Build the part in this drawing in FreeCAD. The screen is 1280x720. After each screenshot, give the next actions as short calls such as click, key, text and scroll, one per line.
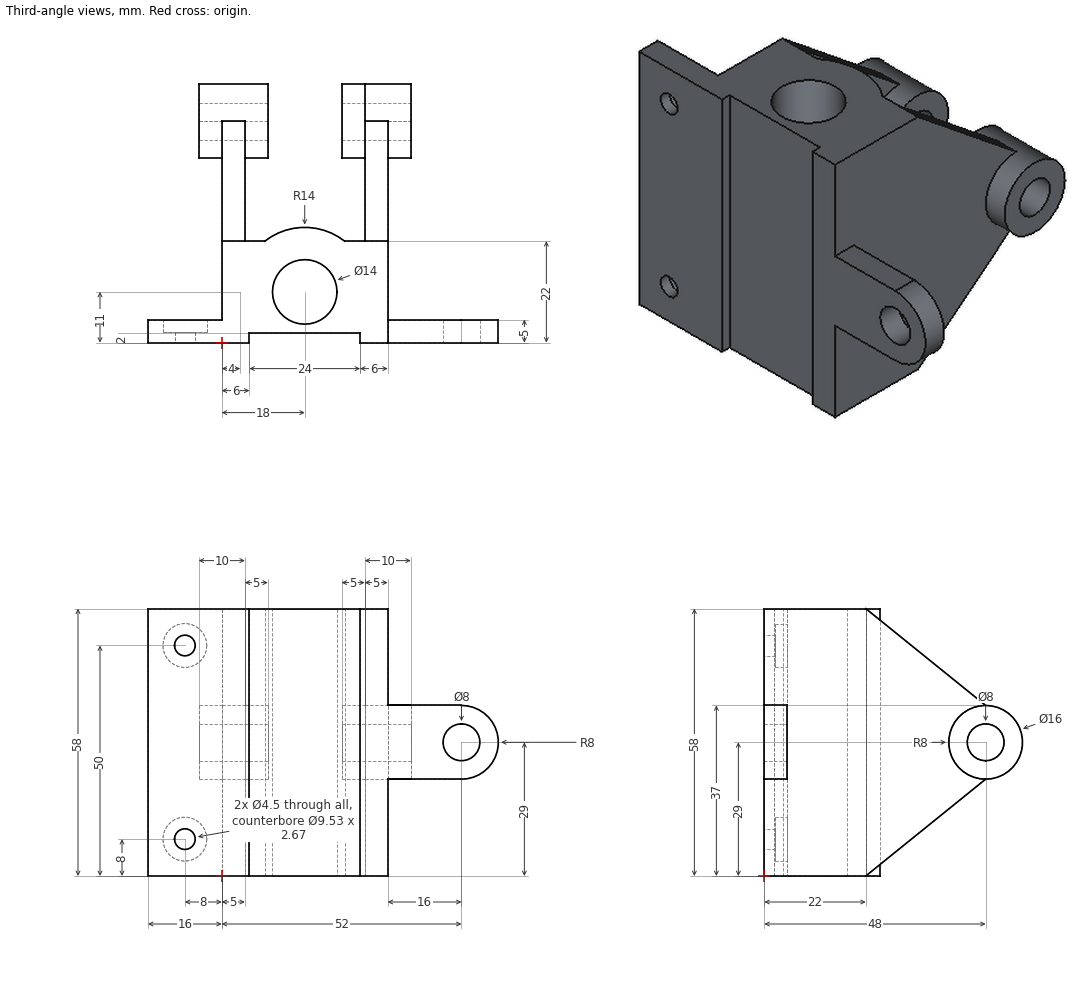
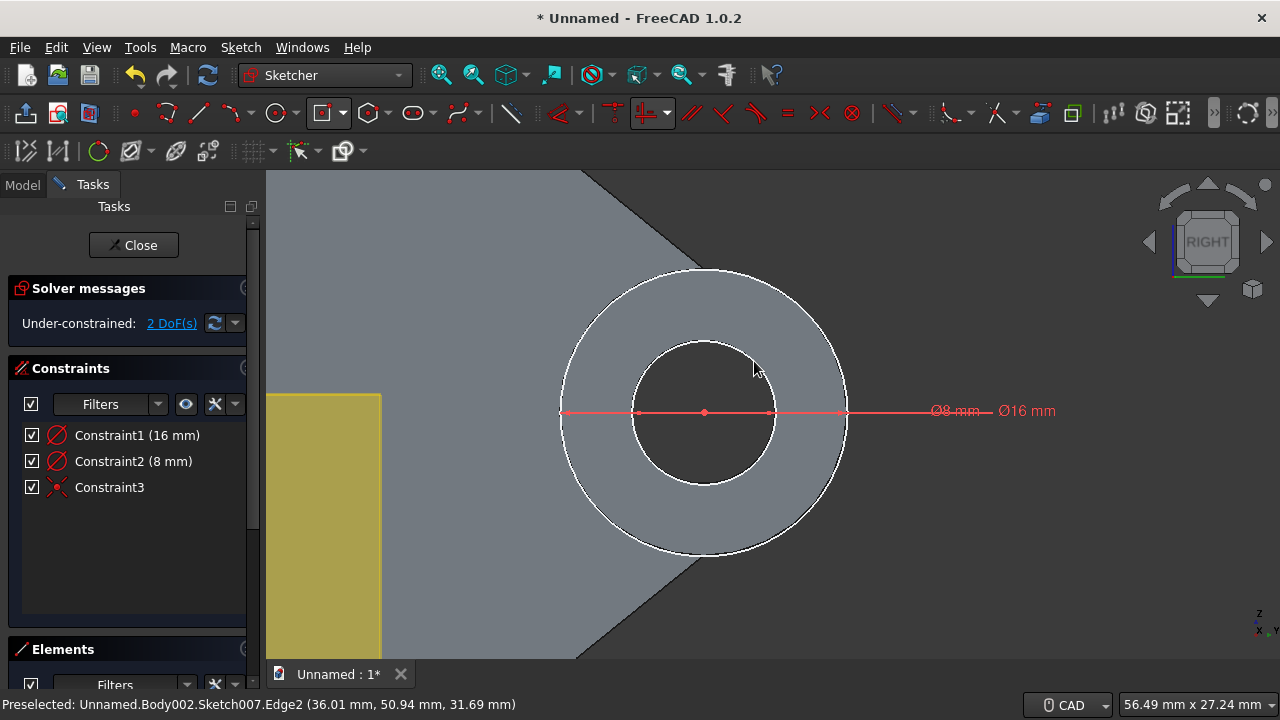
key(d)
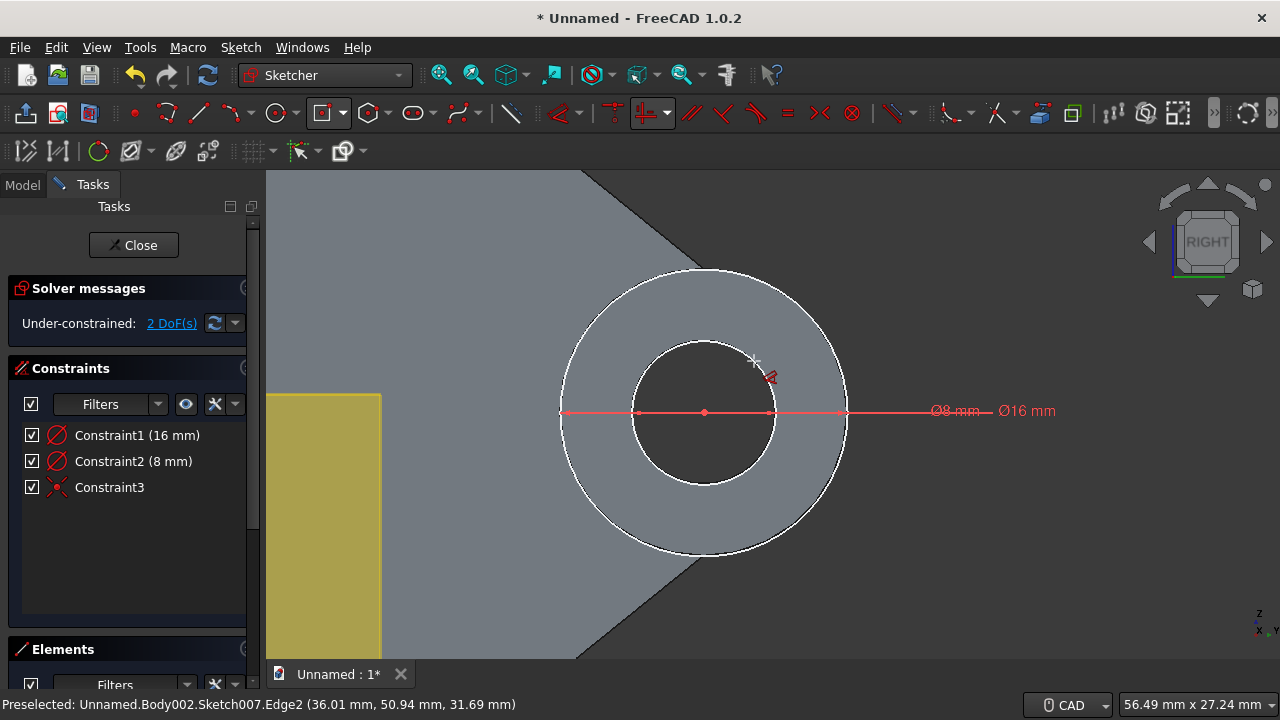
click(704, 413)
click(499, 379)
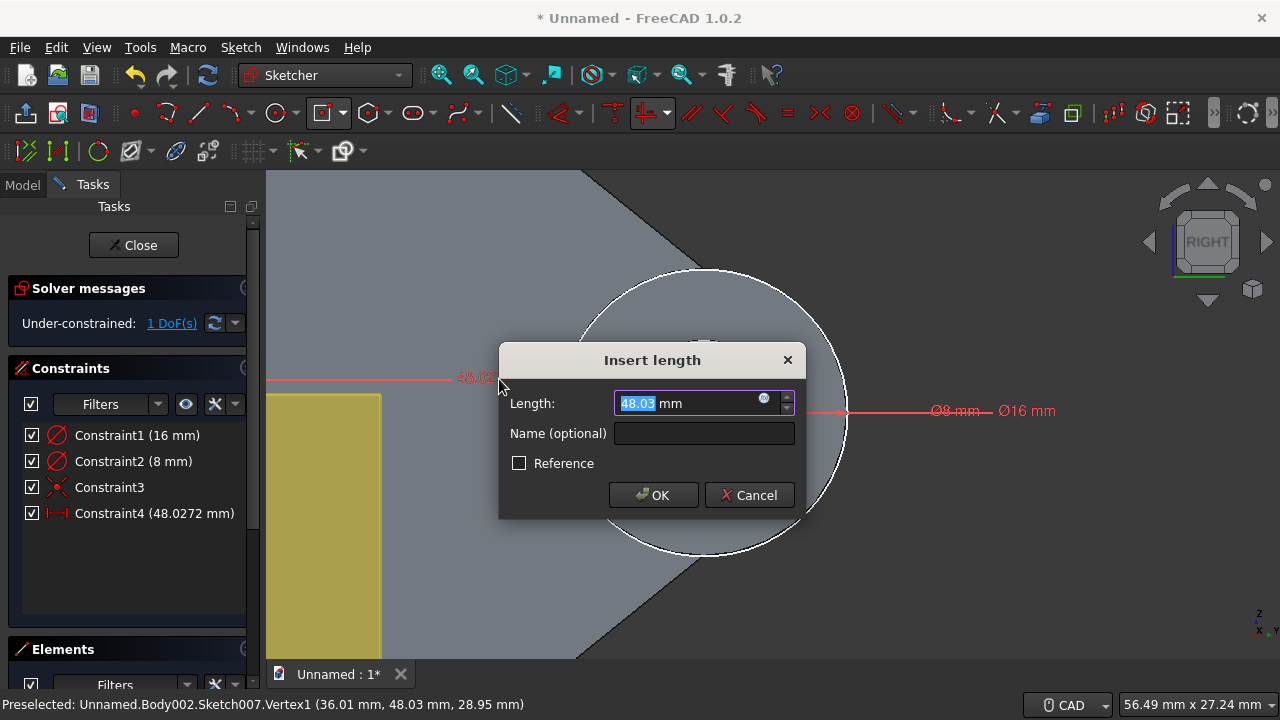
text(48)
key(Return)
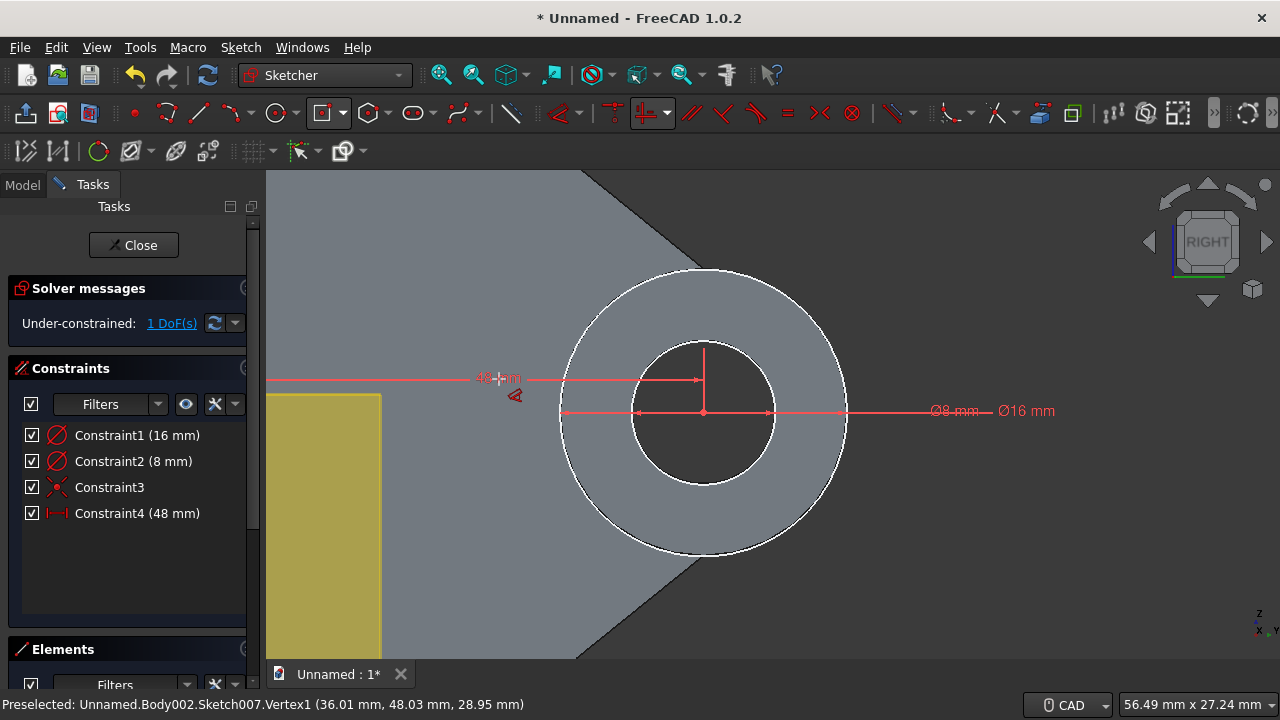
click(704, 413)
click(738, 522)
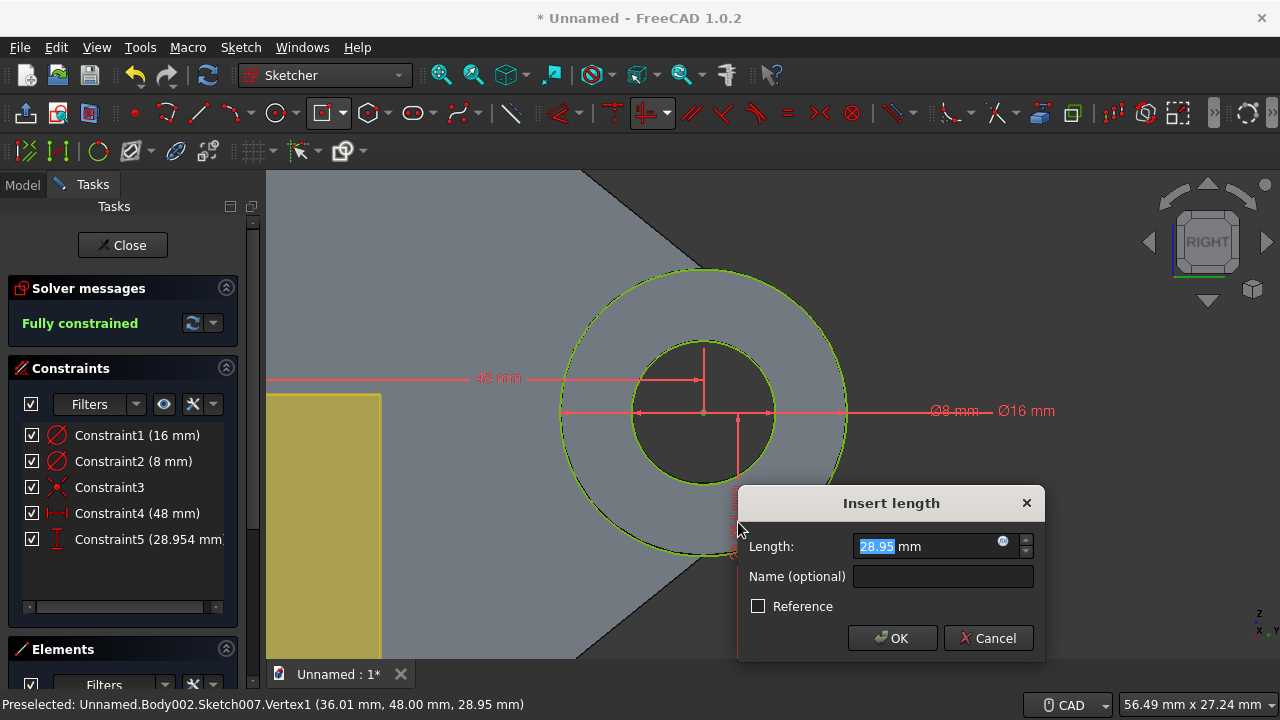
text(29)
key(Return)
key(Escape)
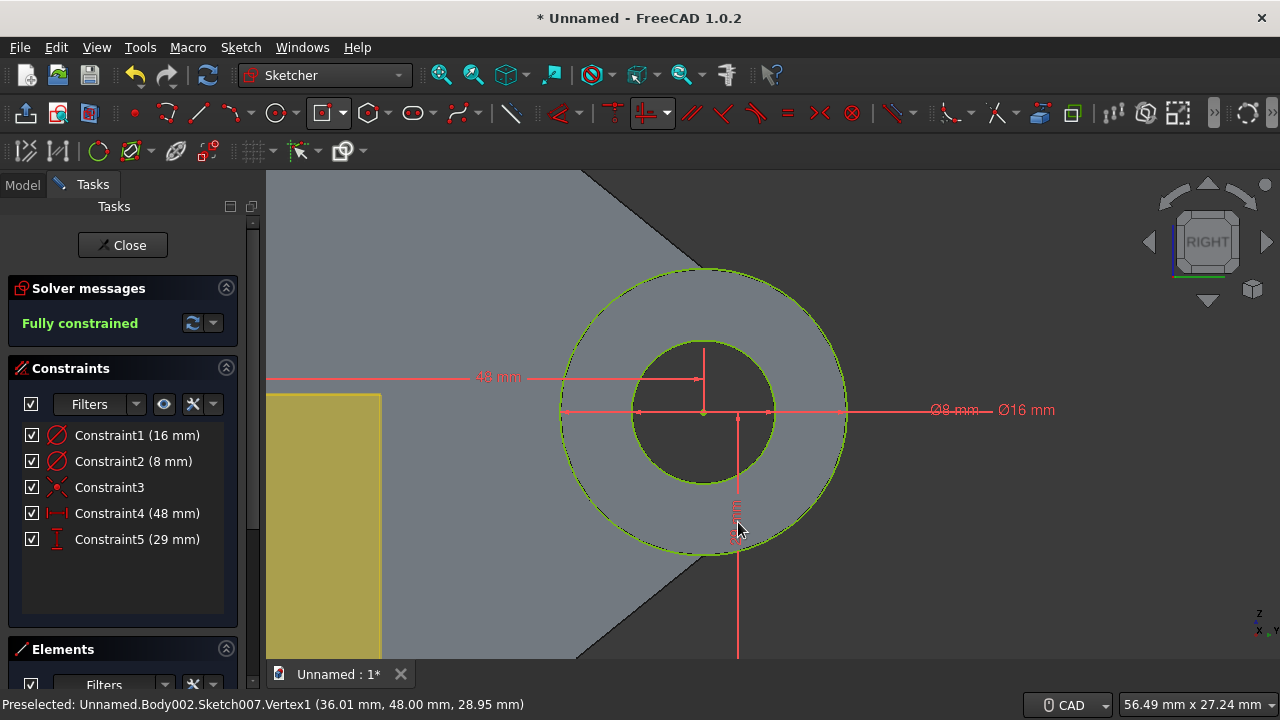
click(123, 245)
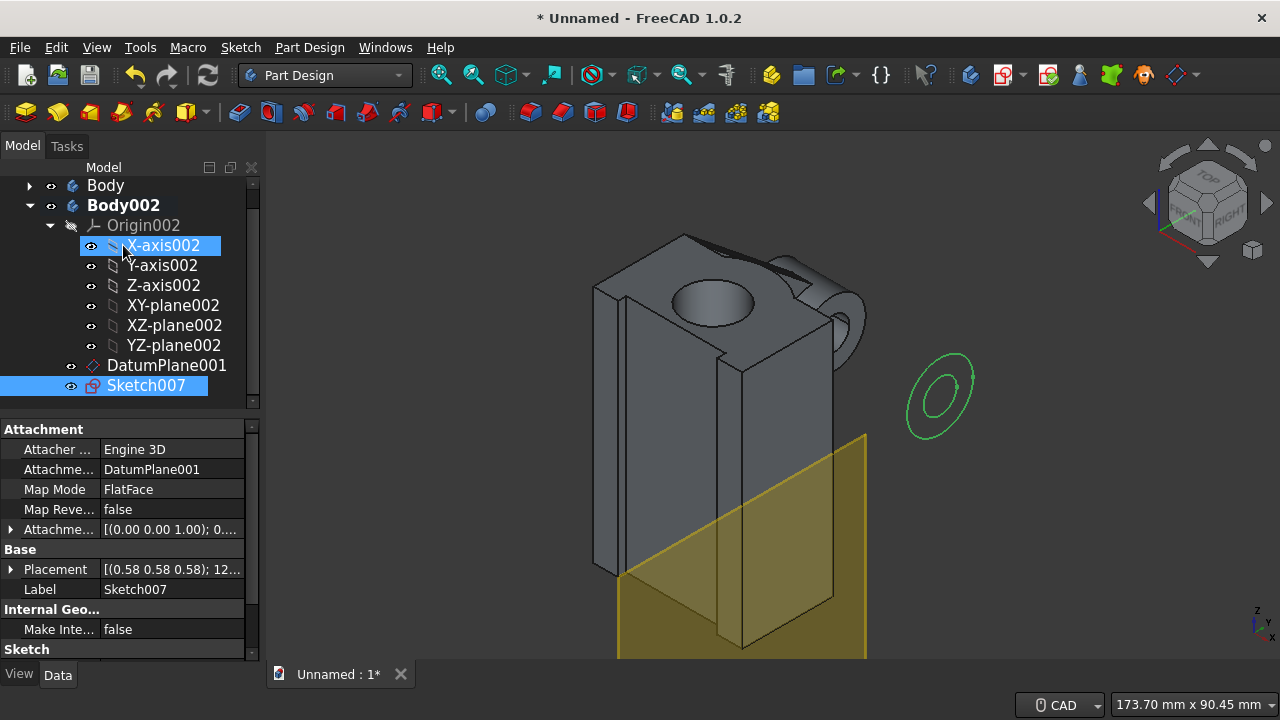
click(26, 112)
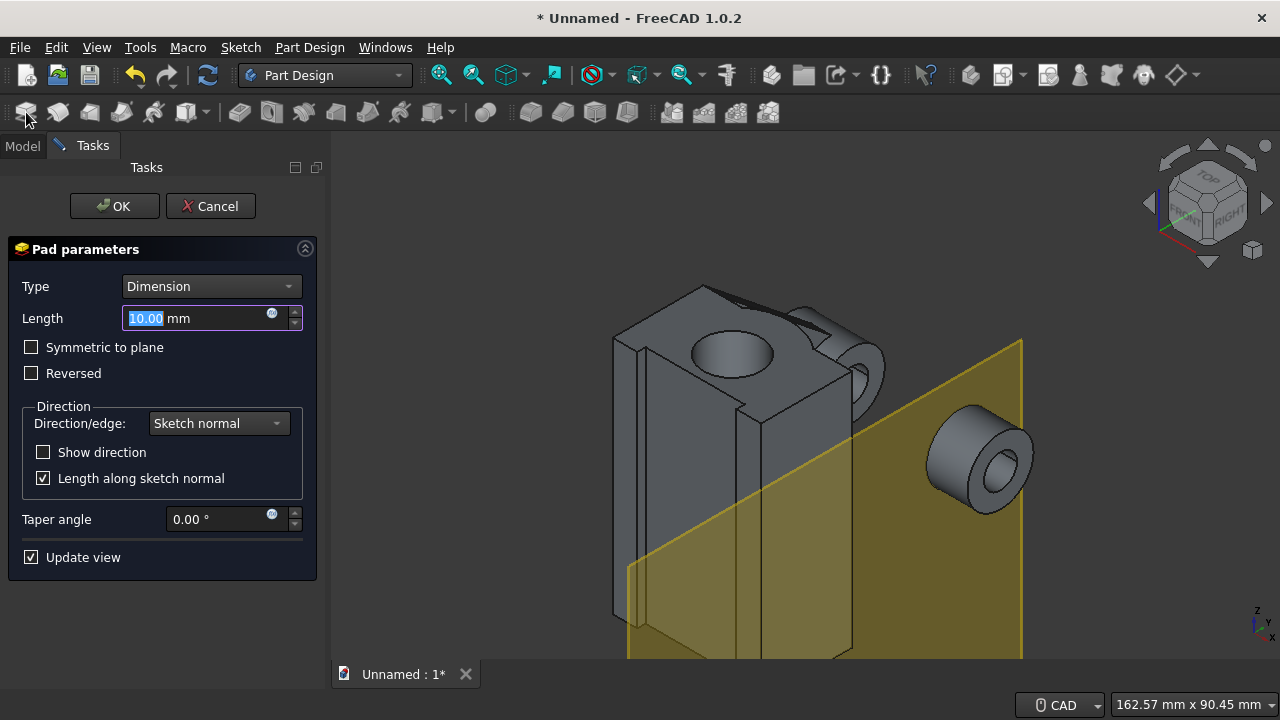
text(10)
key(Tab)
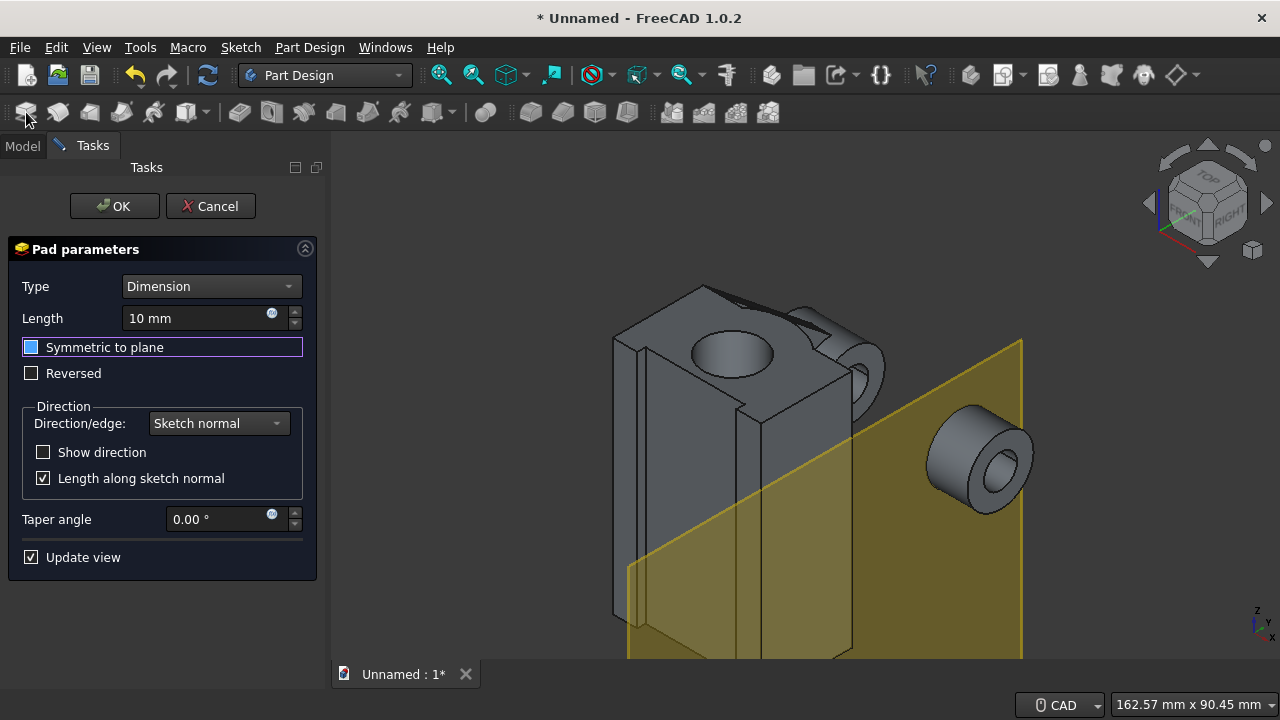
click(30, 347)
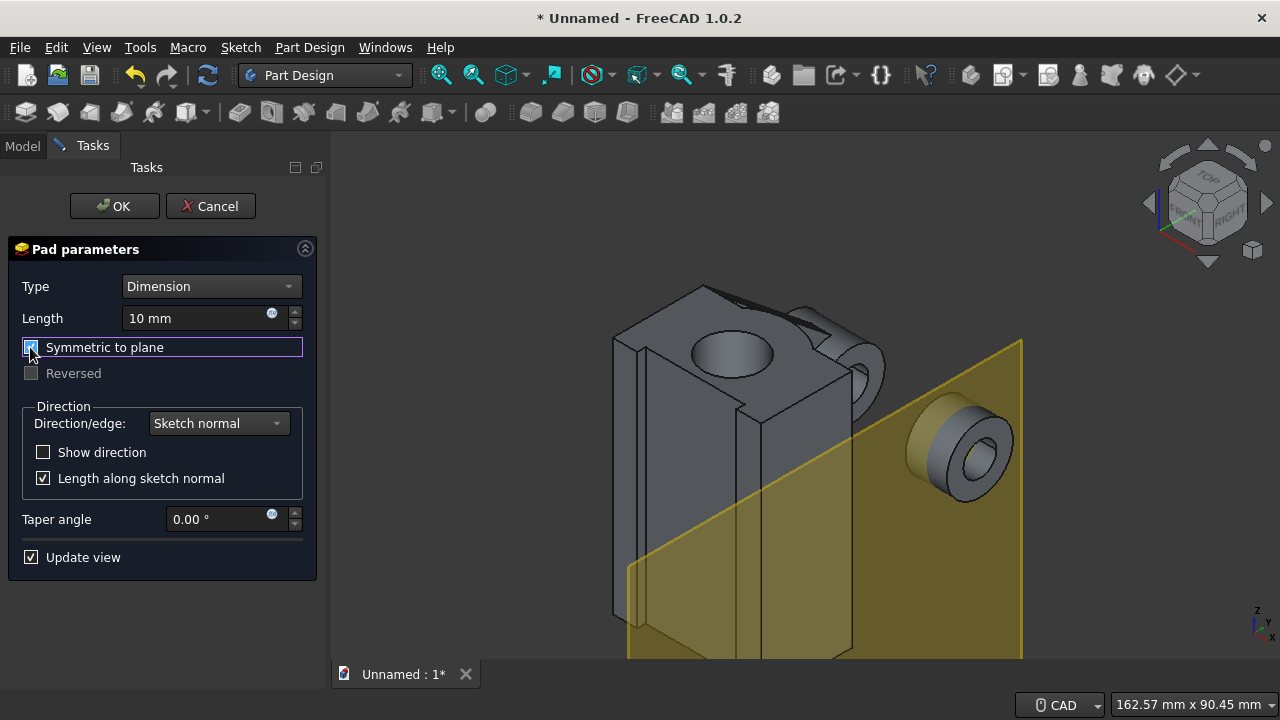
click(115, 206)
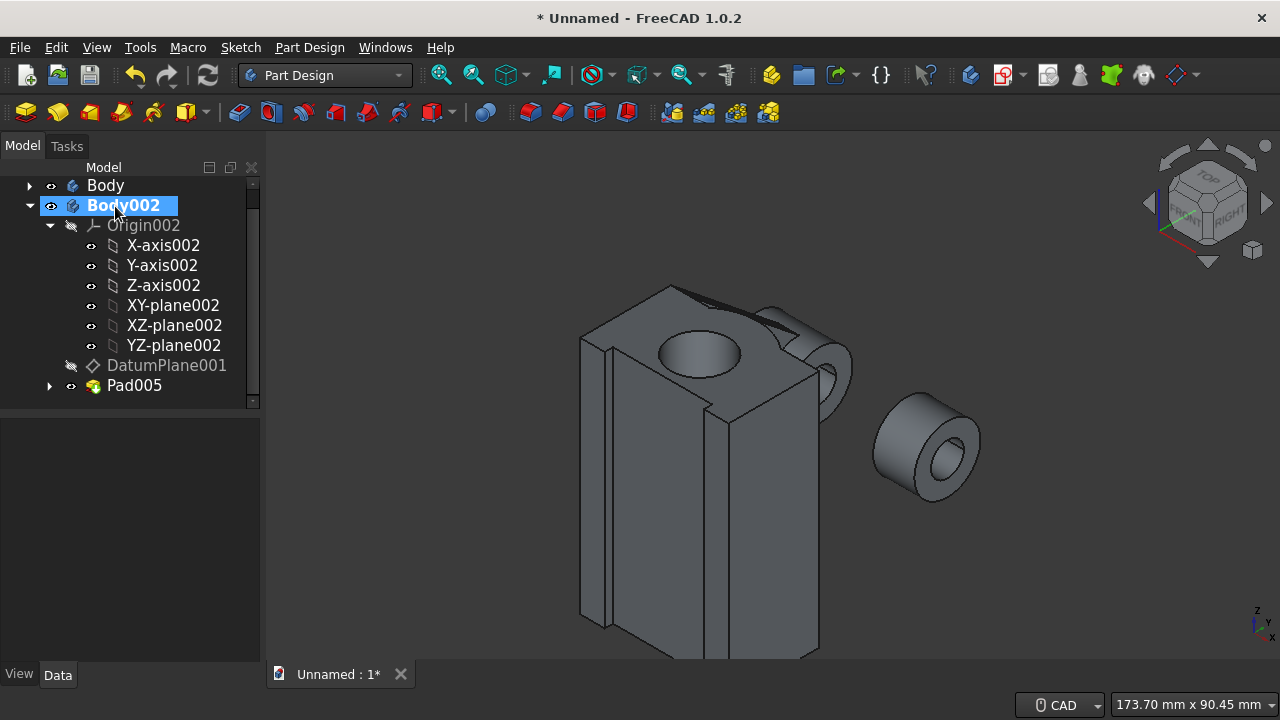
key(v)
key(f)